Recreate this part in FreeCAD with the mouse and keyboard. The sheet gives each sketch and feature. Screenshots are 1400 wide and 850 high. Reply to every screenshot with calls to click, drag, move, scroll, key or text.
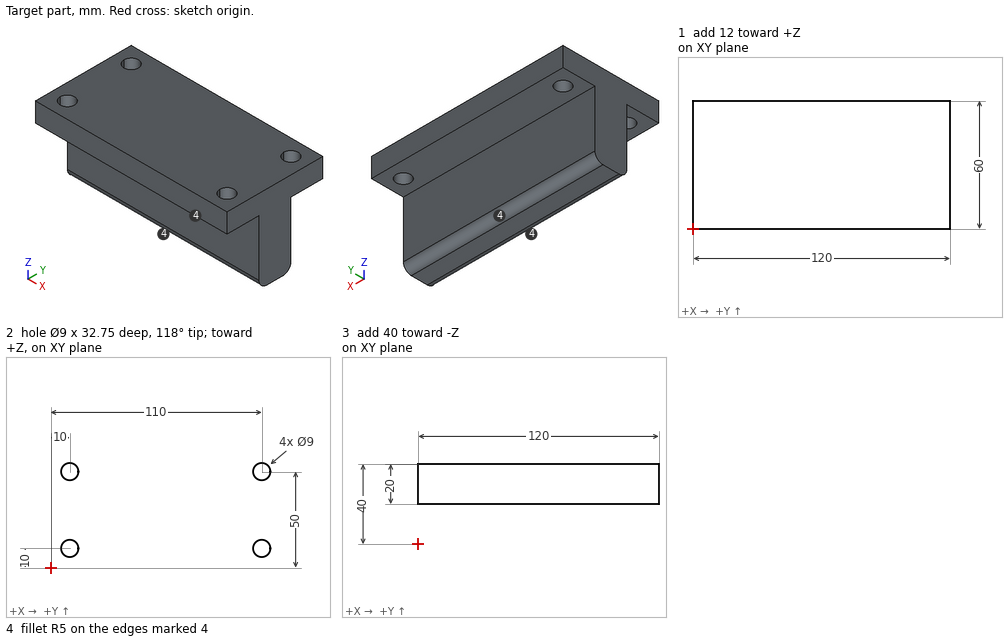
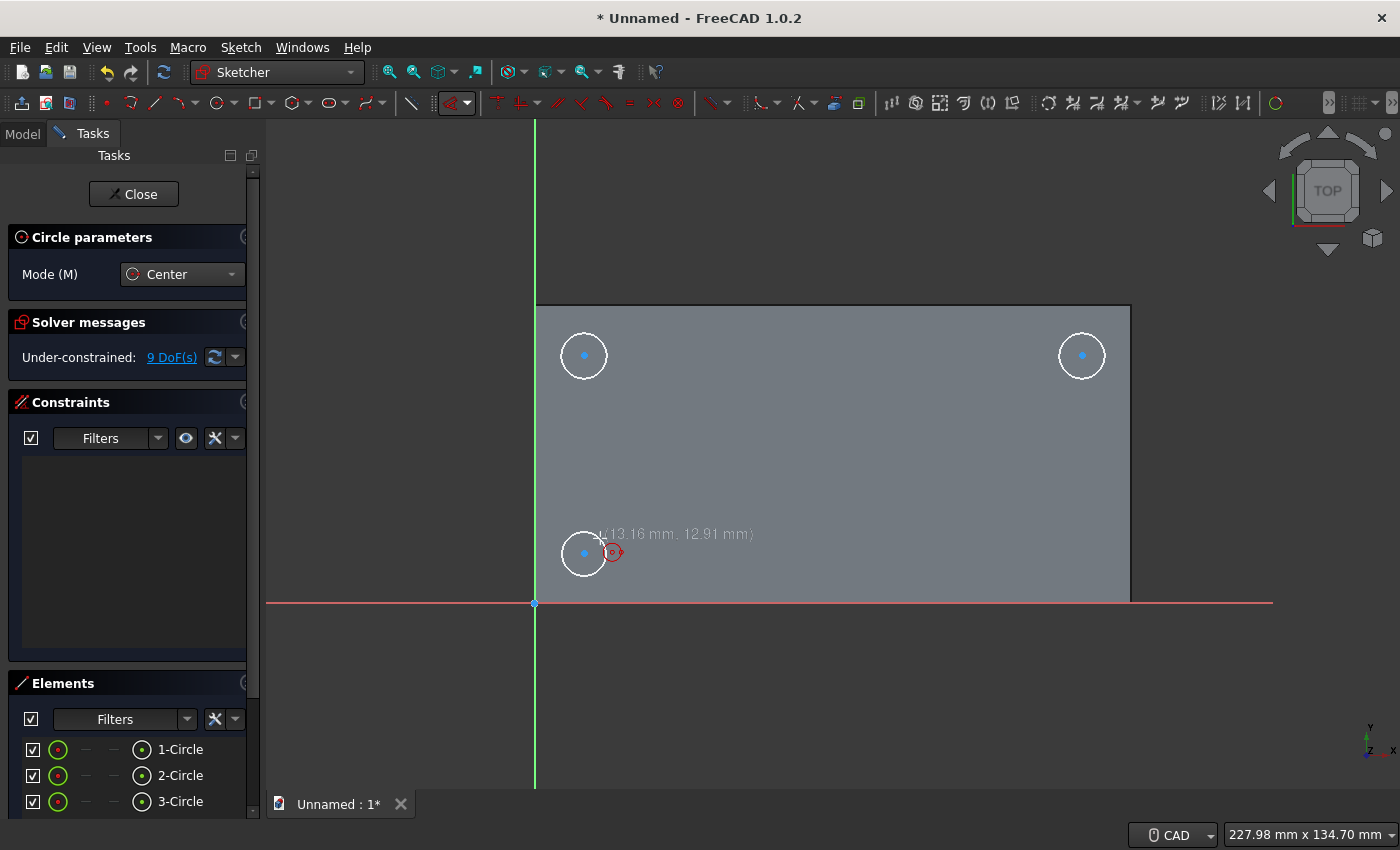
click(1082, 553)
click(1098, 538)
key(Escape)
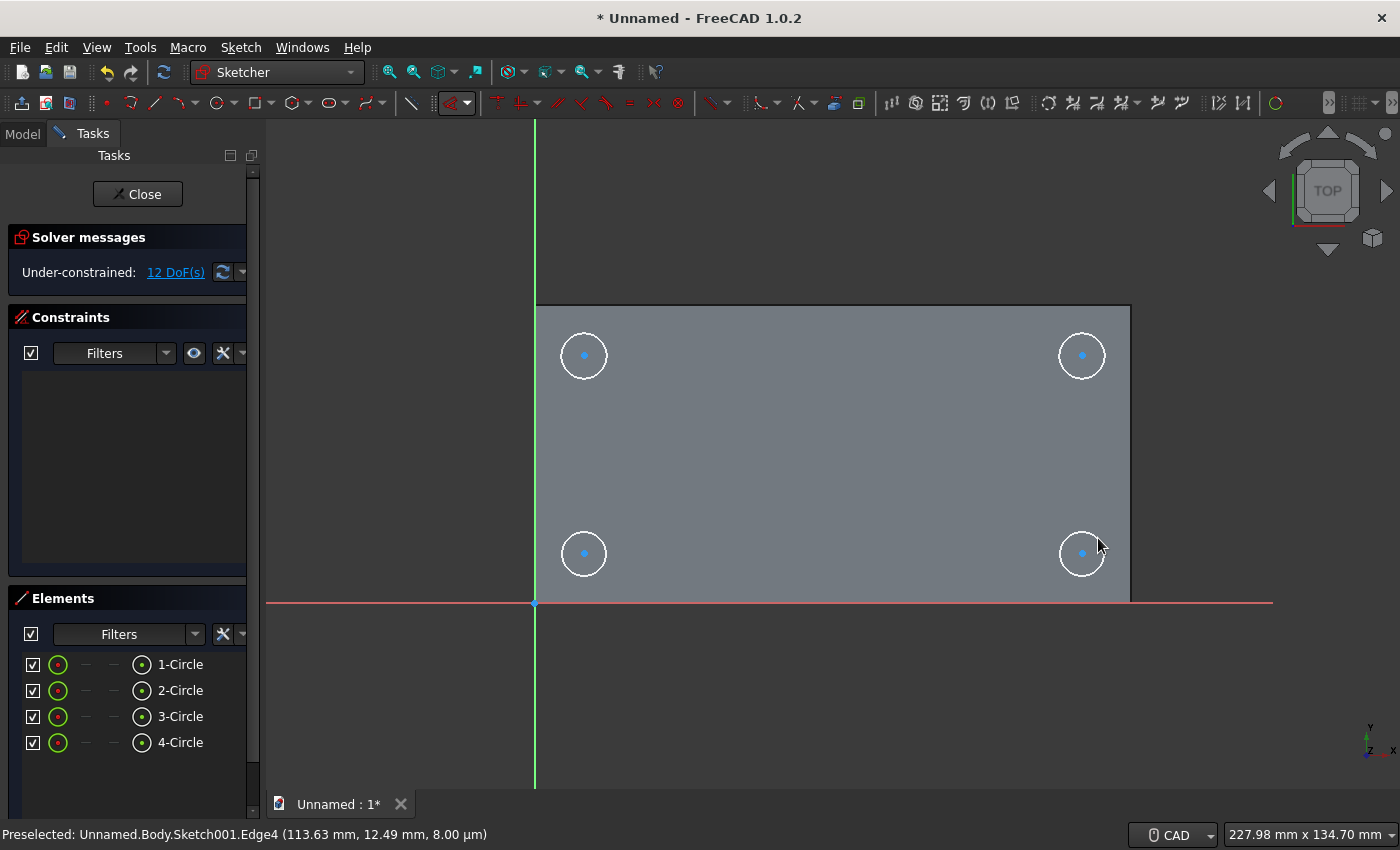
click(1098, 340)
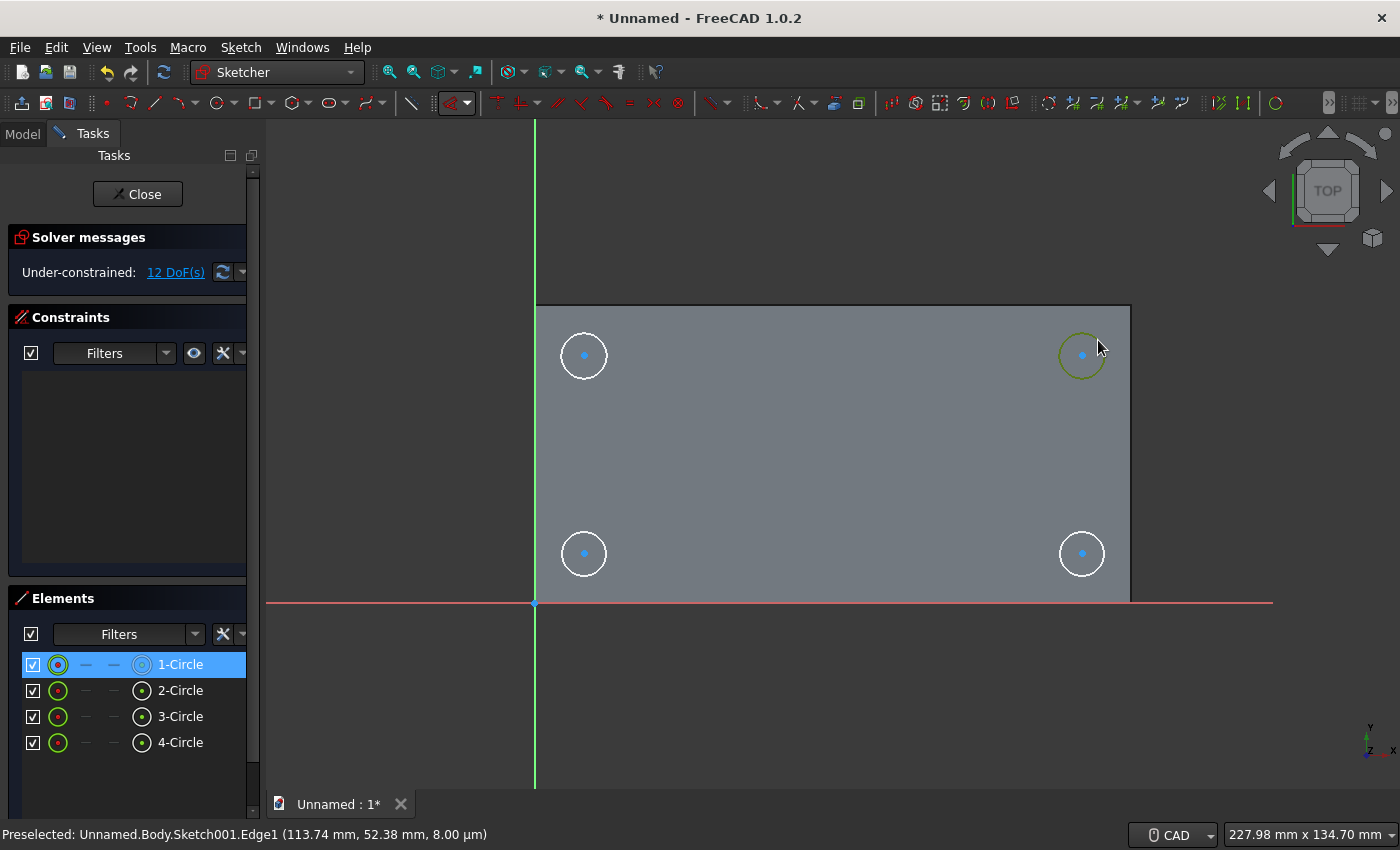
click(600, 340)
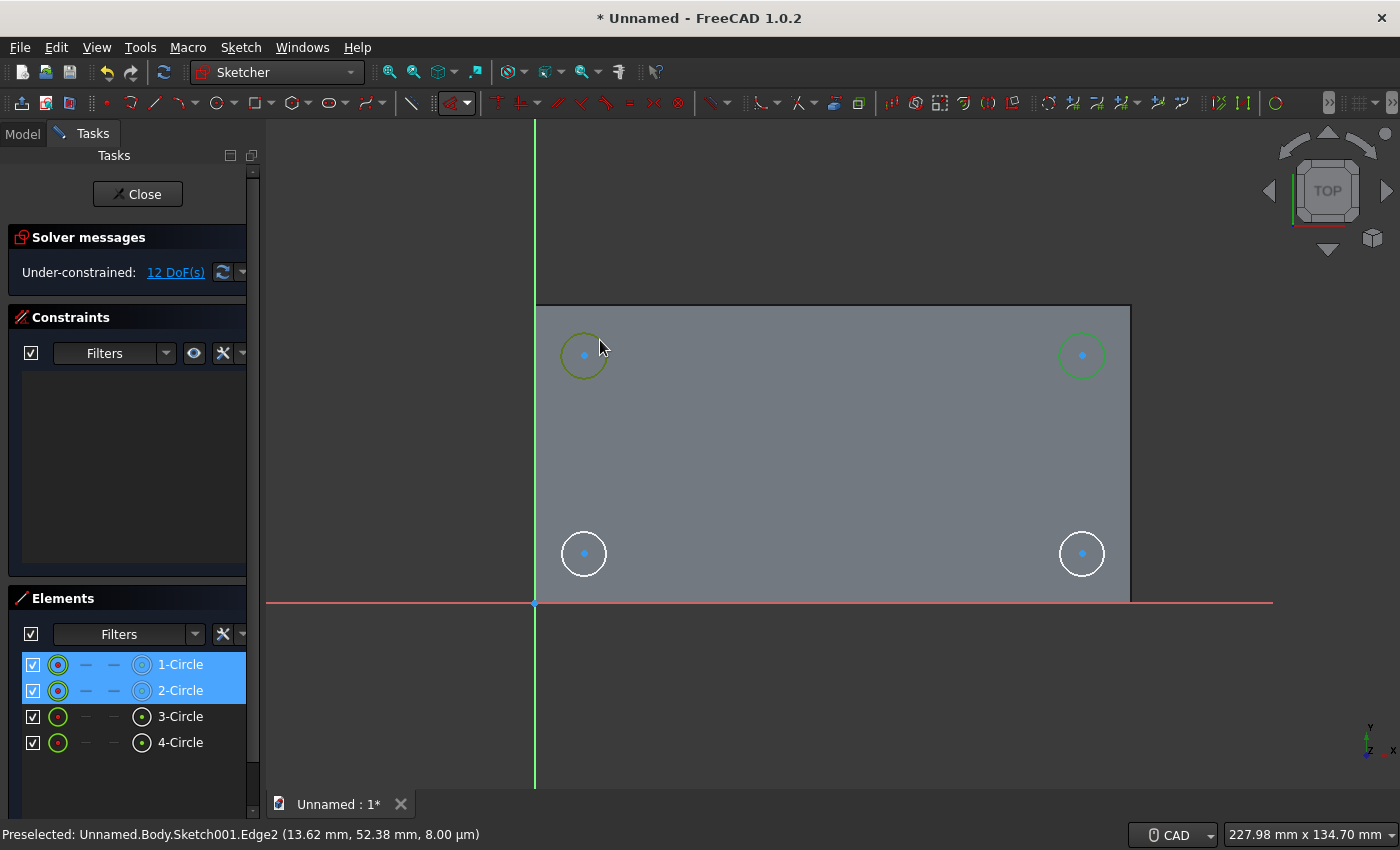
click(599, 538)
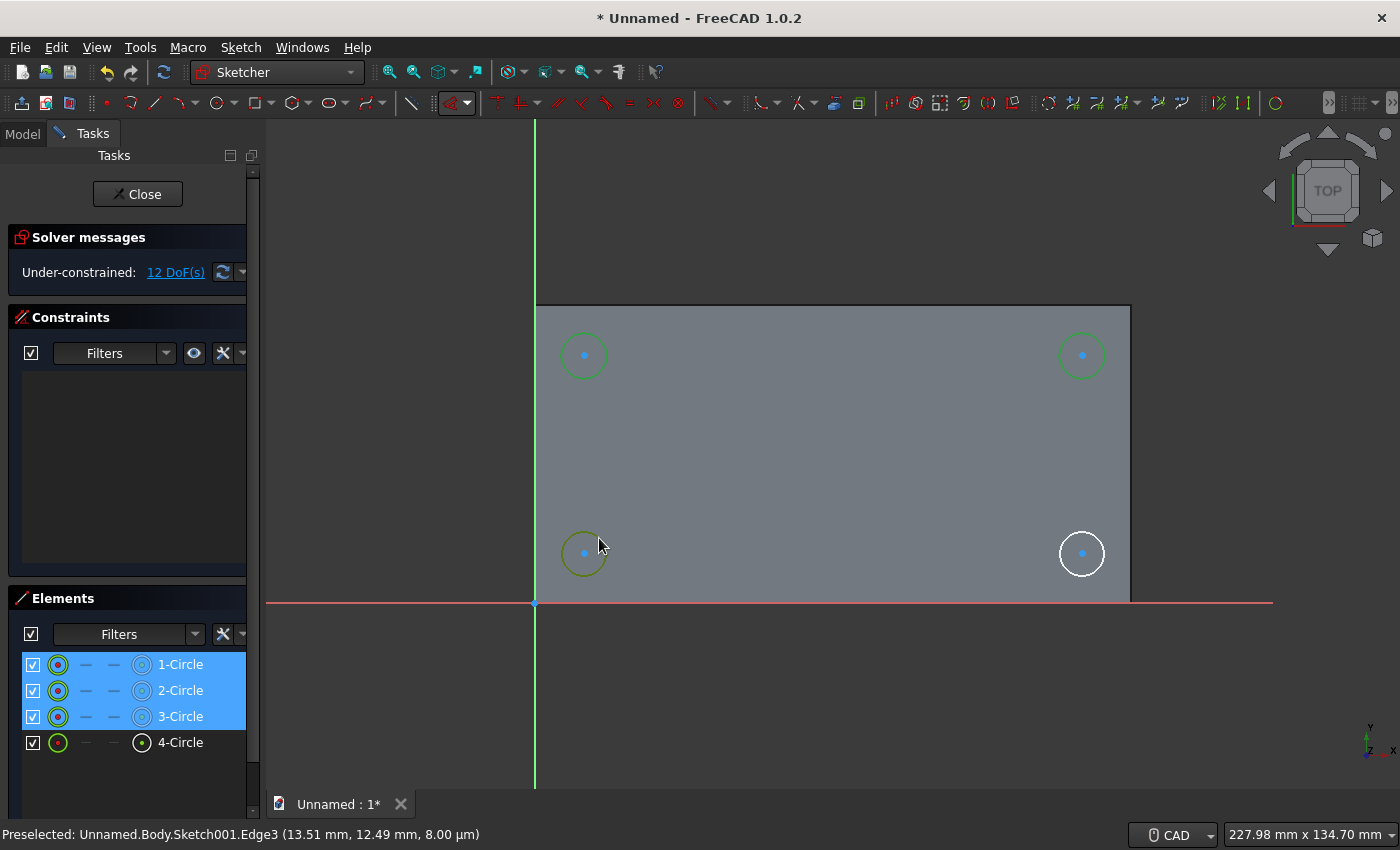
click(1097, 538)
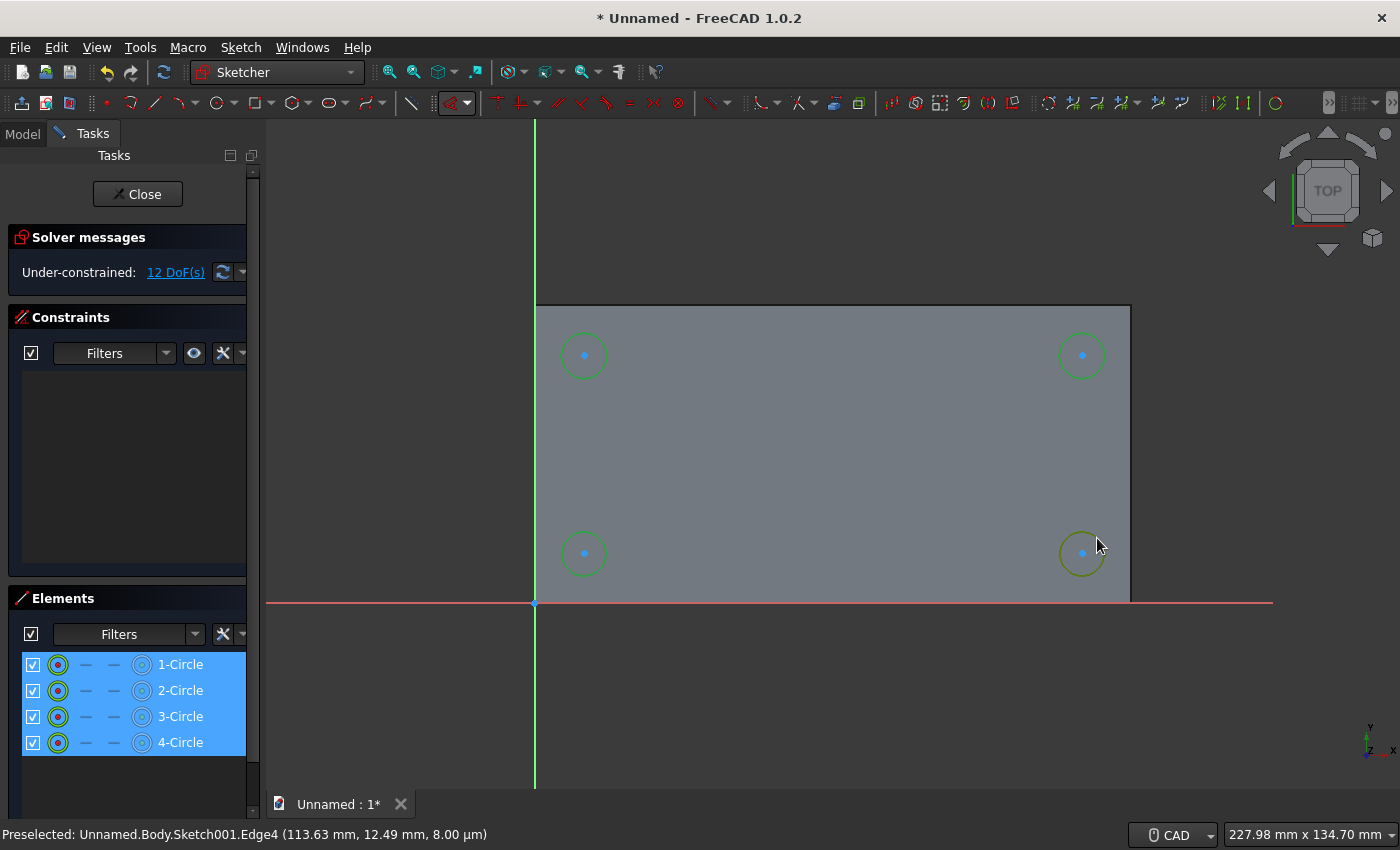
click(630, 104)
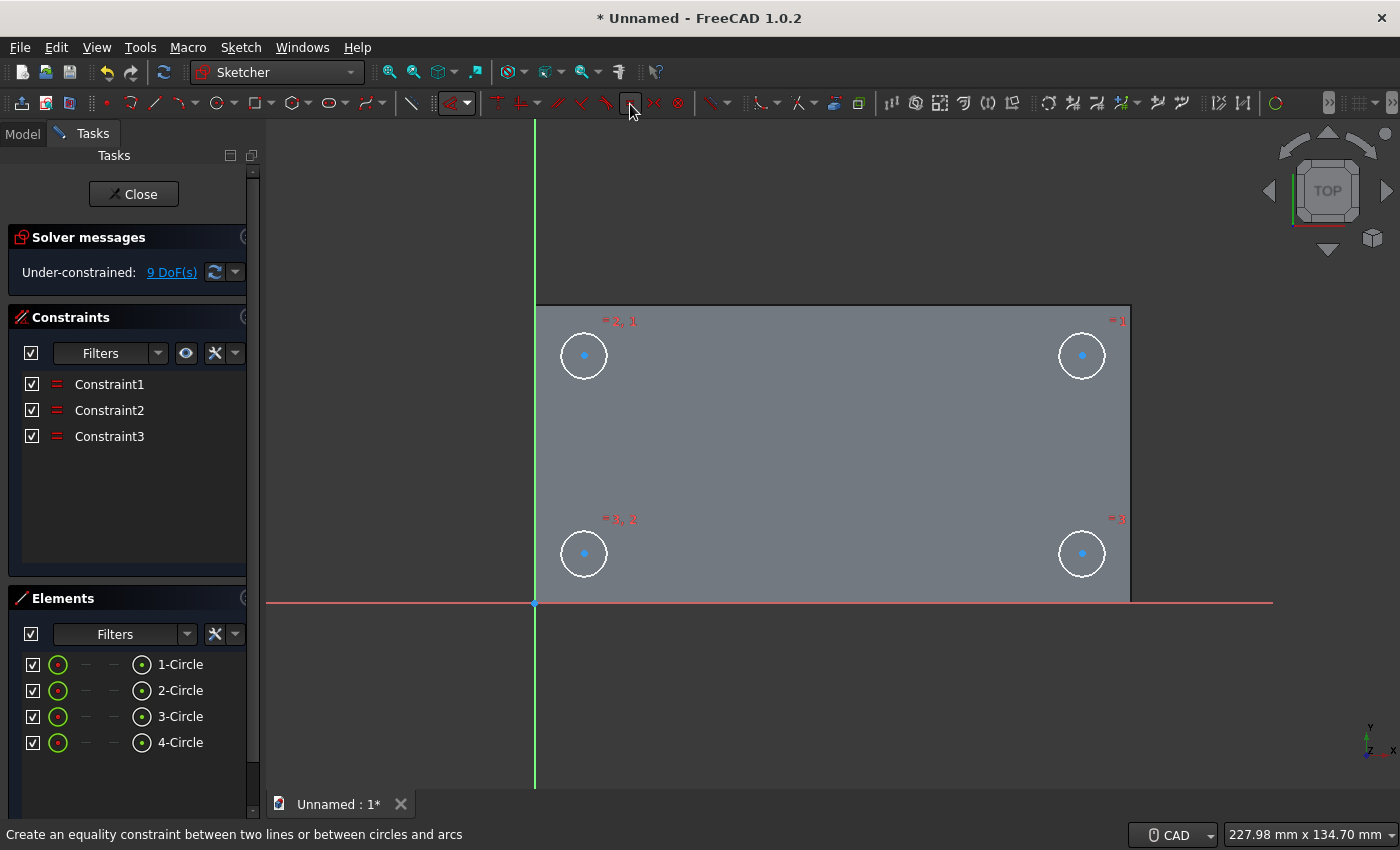
click(1082, 356)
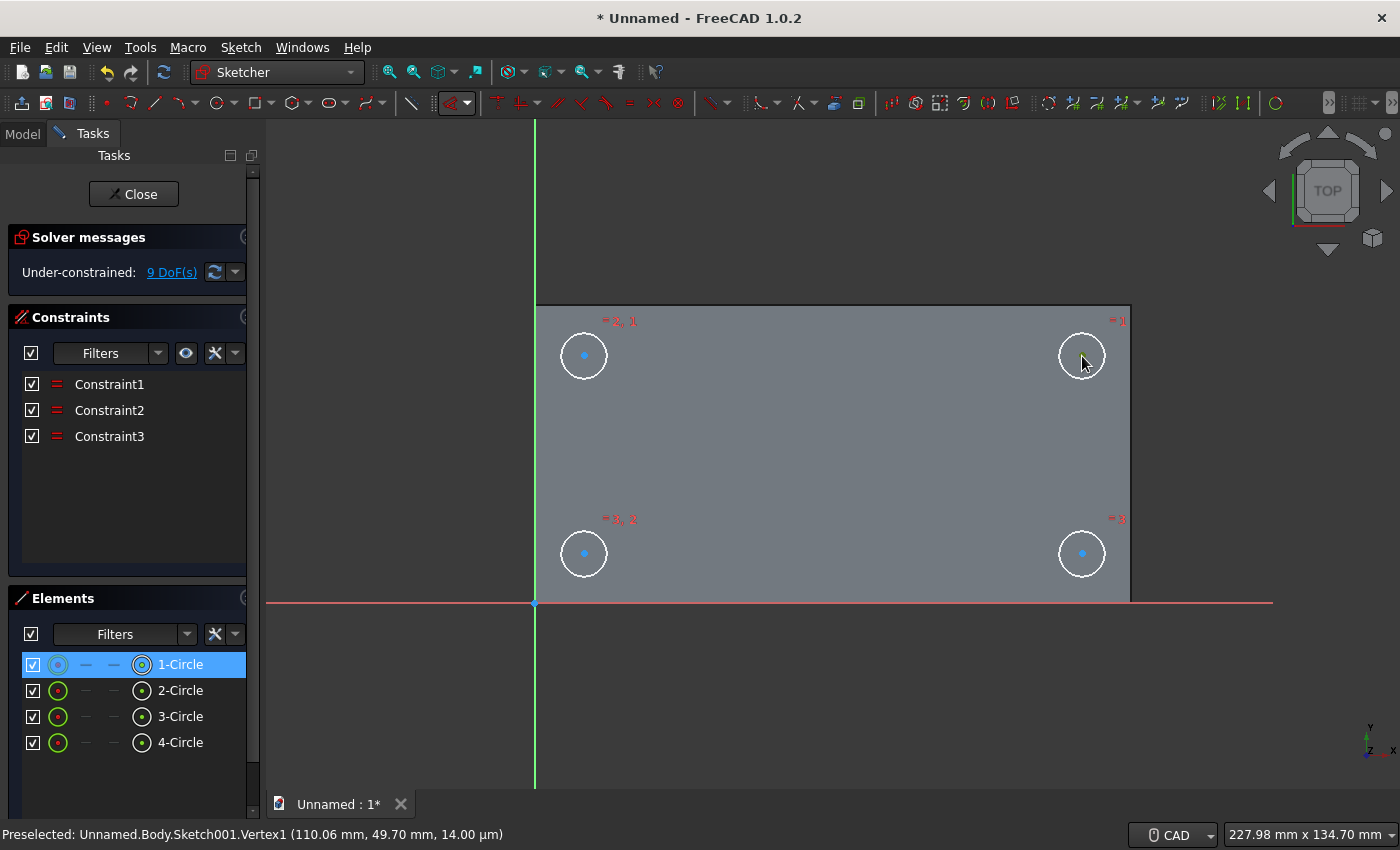
click(584, 356)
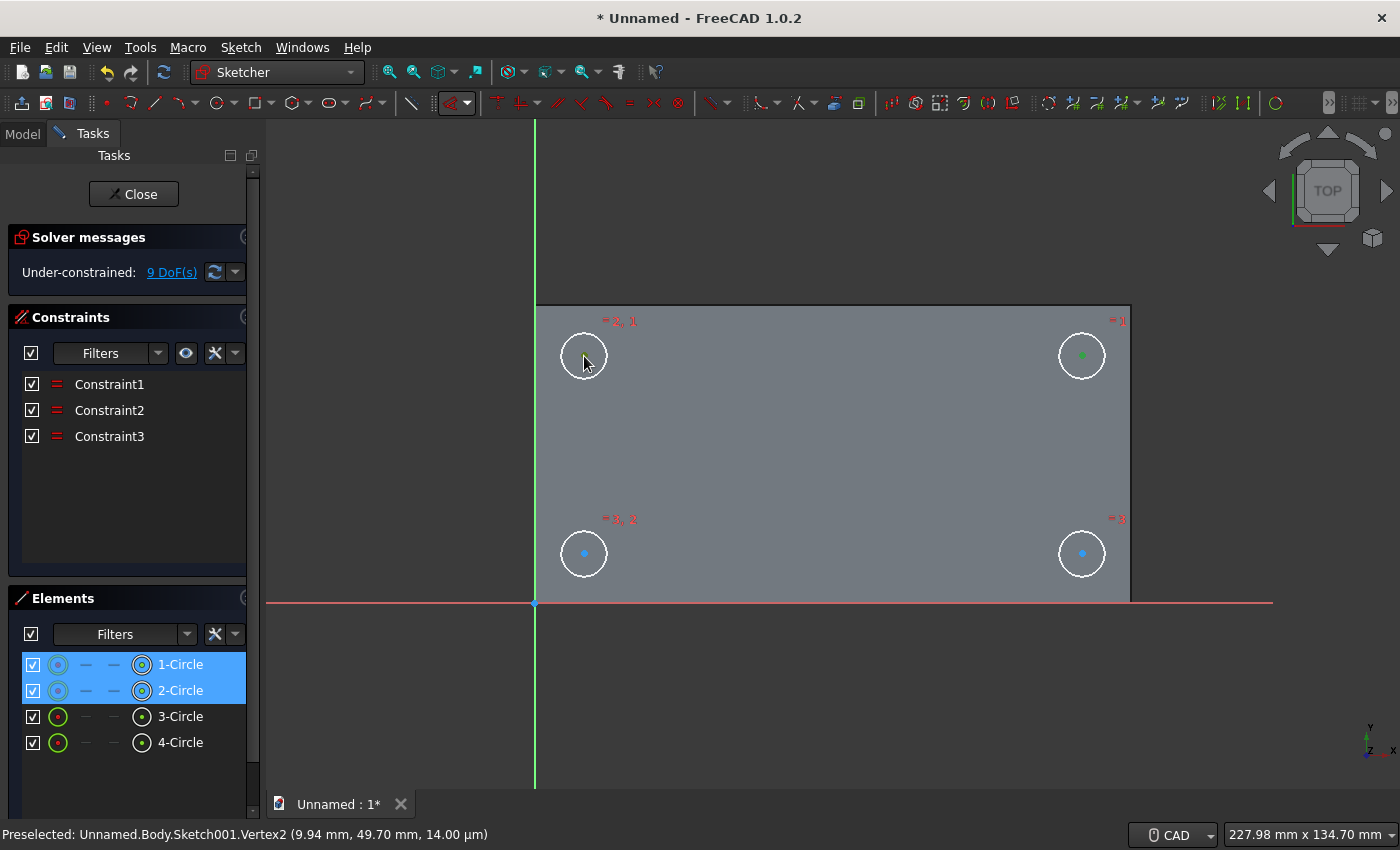
click(540, 104)